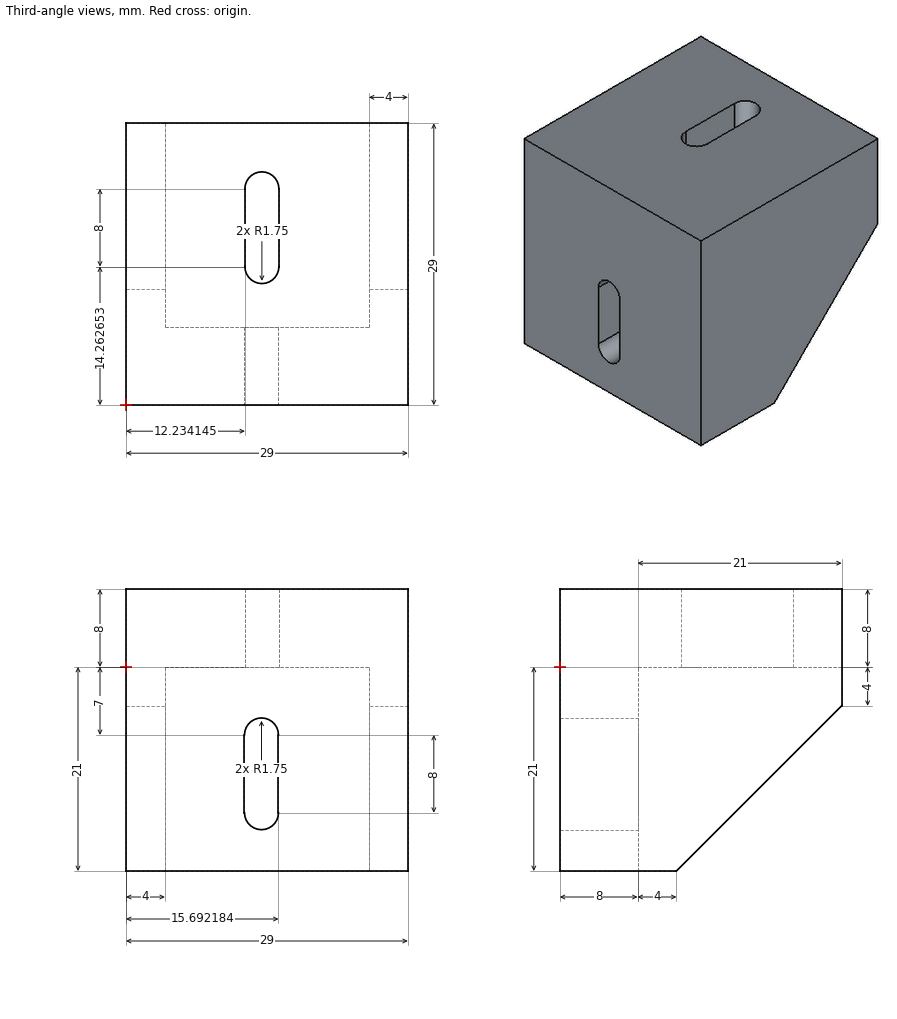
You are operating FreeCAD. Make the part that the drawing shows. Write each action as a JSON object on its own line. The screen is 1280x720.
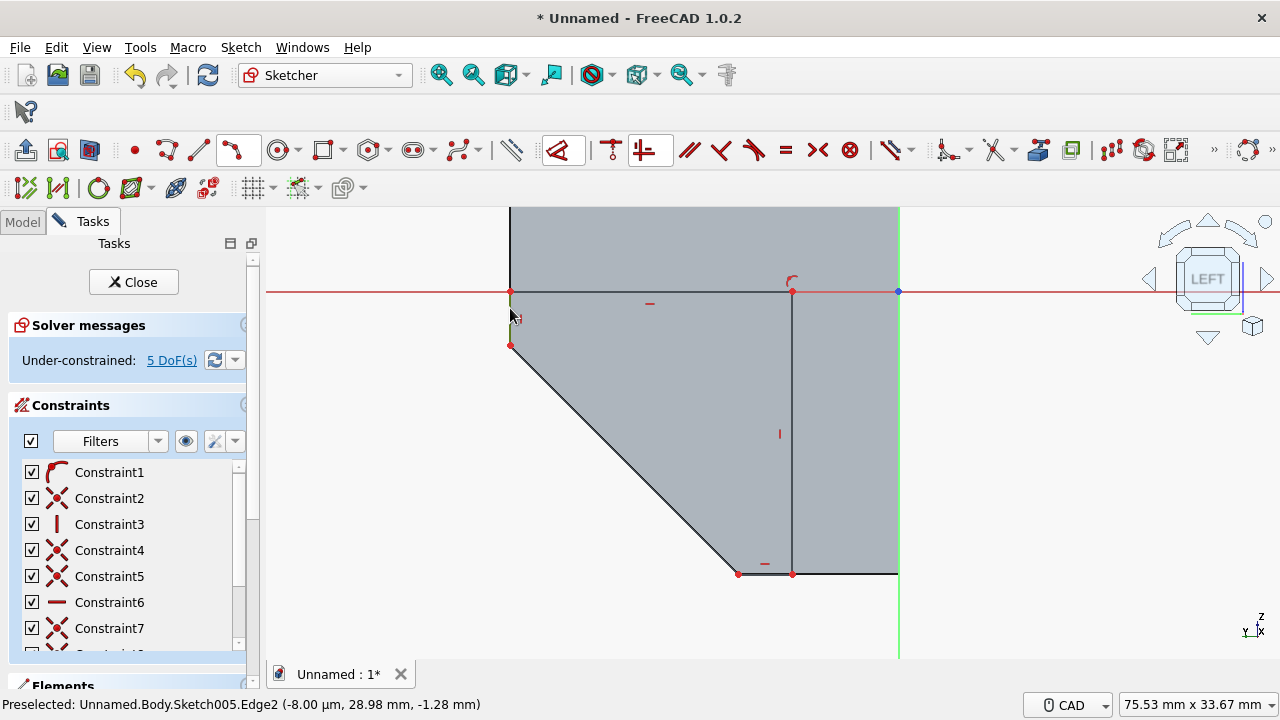
{"action": "key", "text": "i"}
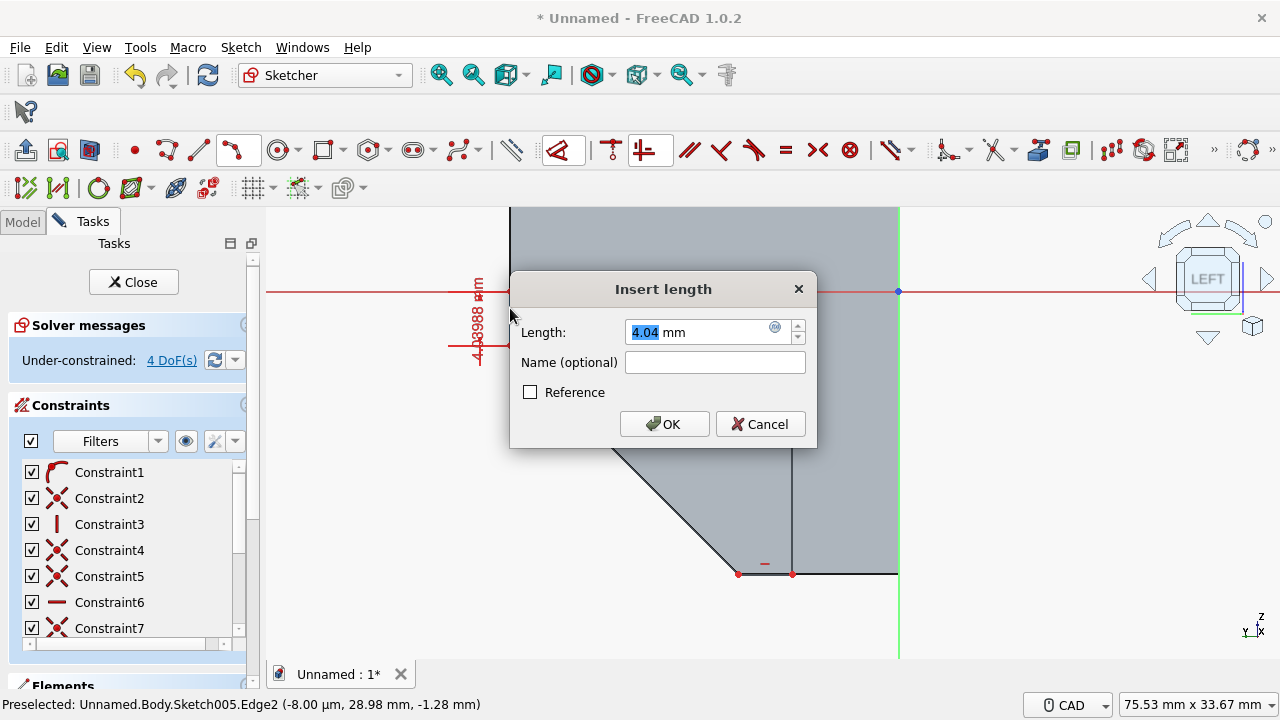
{"action": "type", "text": "4"}
{"action": "key", "text": "Return"}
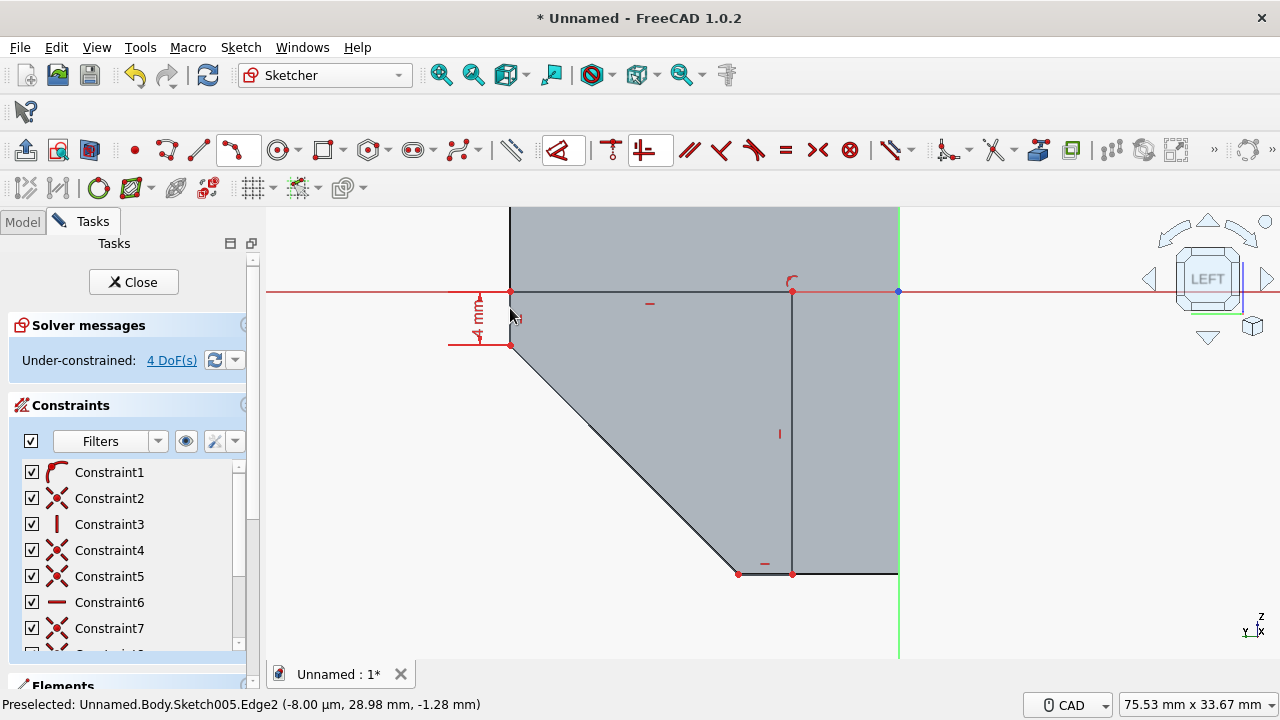
{"action": "left_click", "coordinate": [754, 575]}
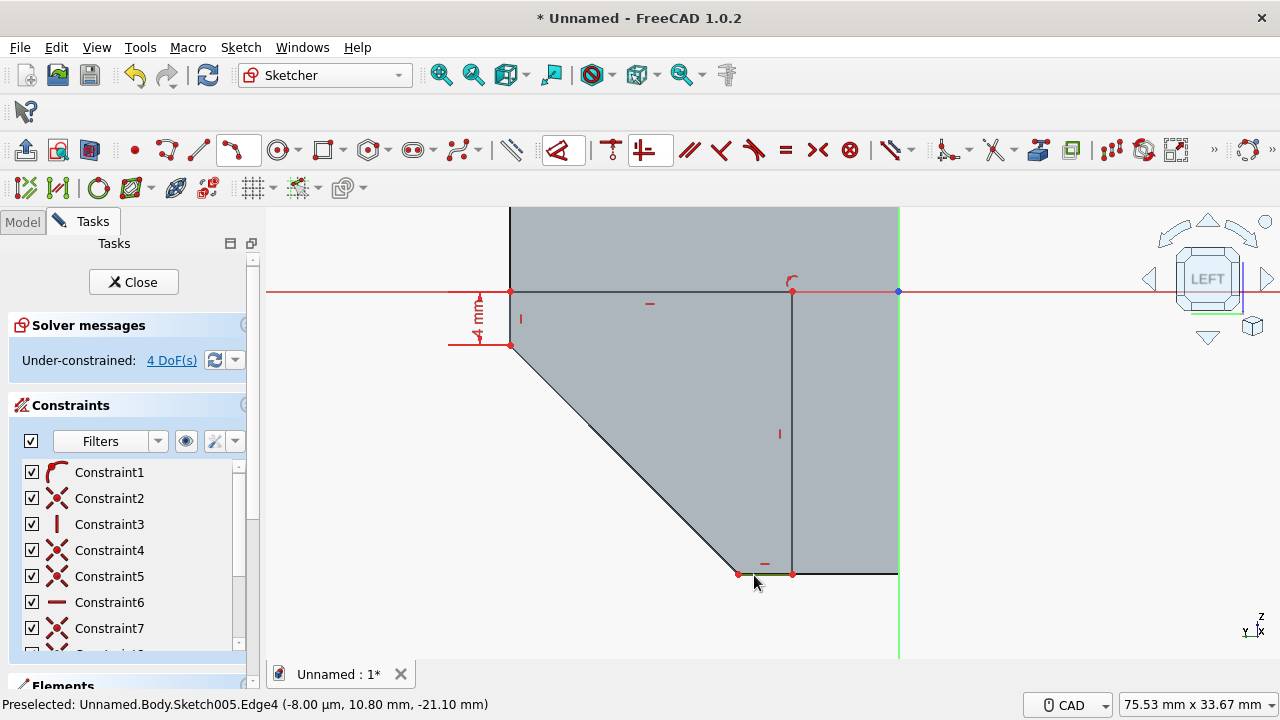
{"action": "left_click", "coordinate": [580, 150]}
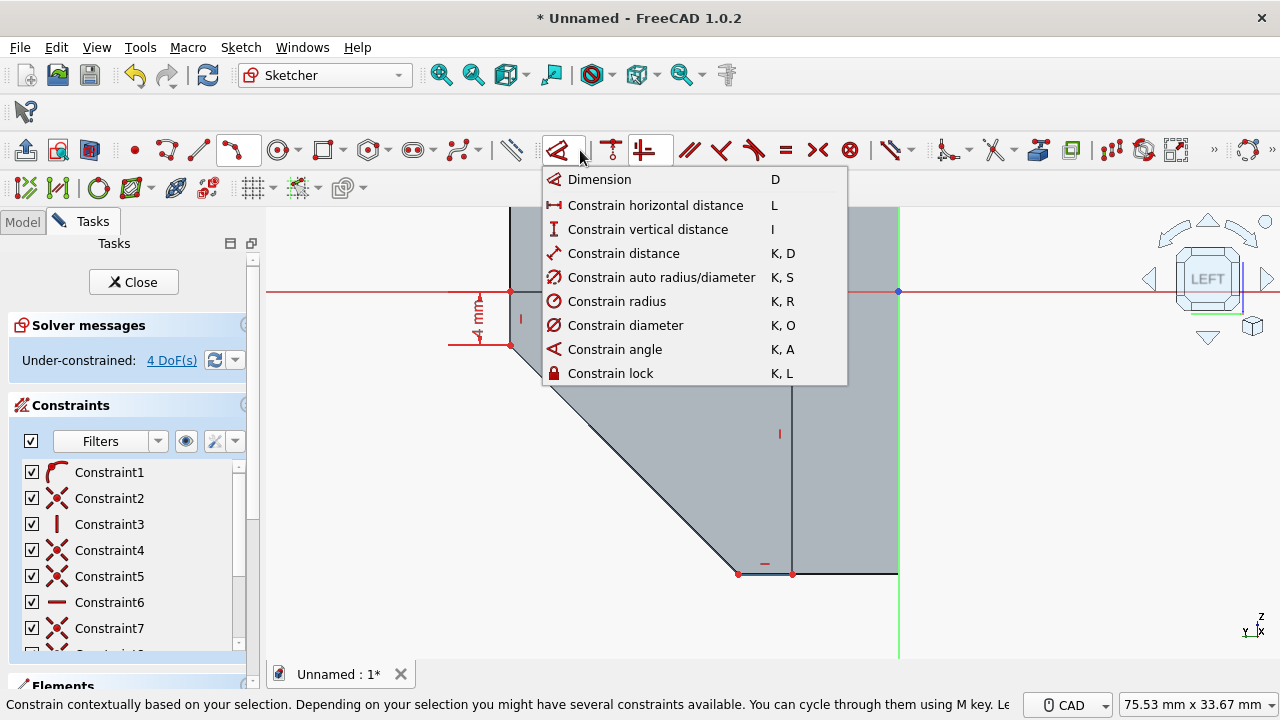
{"action": "left_click", "coordinate": [695, 205]}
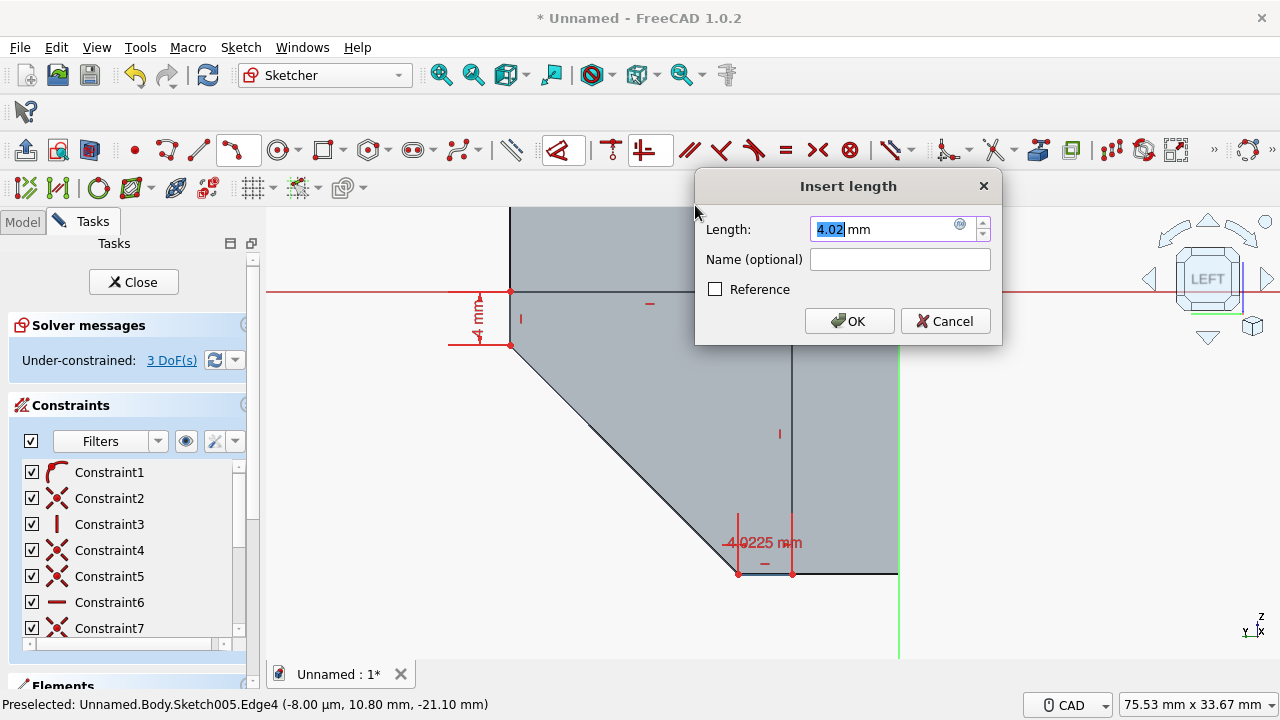
{"action": "type", "text": "4"}
{"action": "key", "text": "Return"}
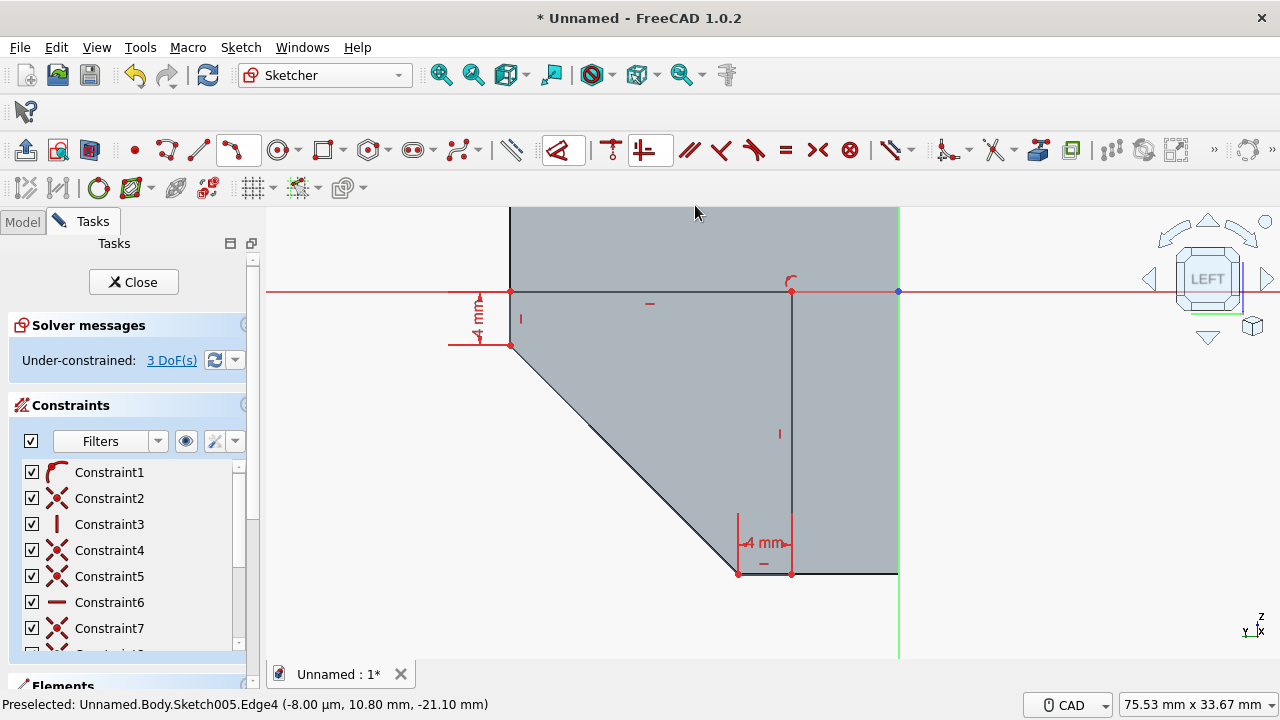
{"action": "left_click", "coordinate": [707, 292]}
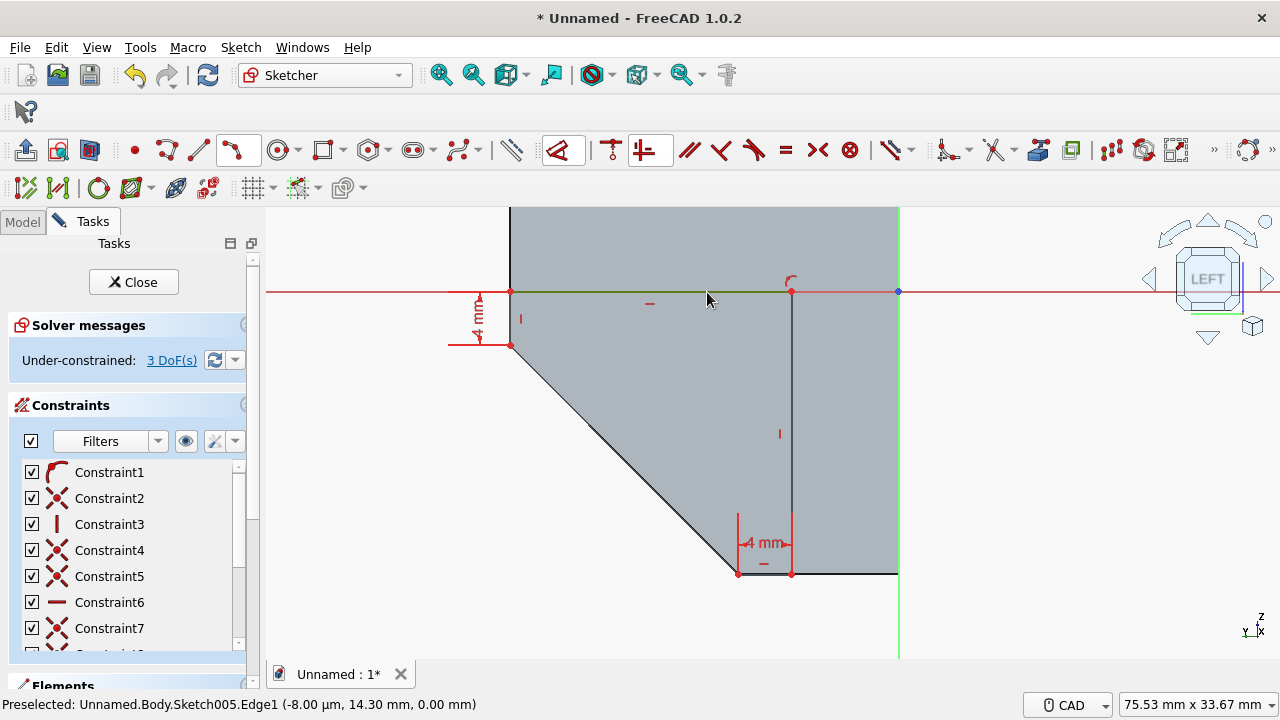
{"action": "key", "text": "l"}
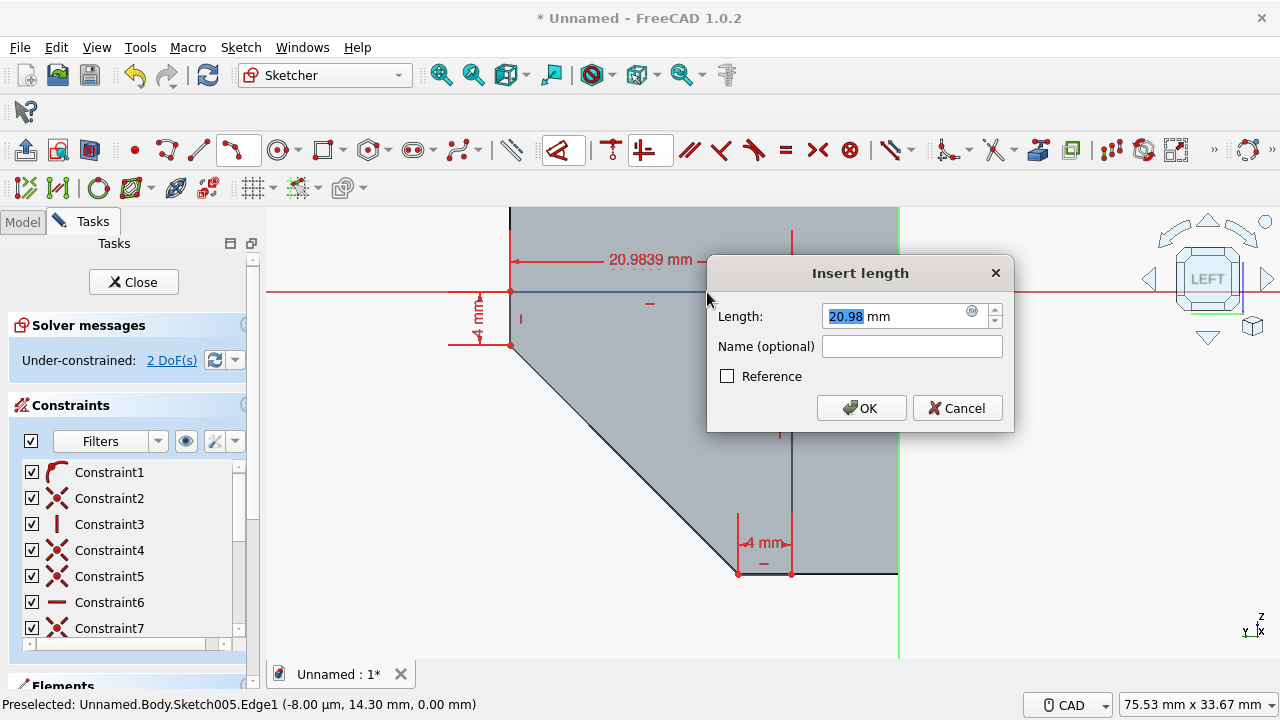
{"action": "type", "text": "21"}
{"action": "key", "text": "Return"}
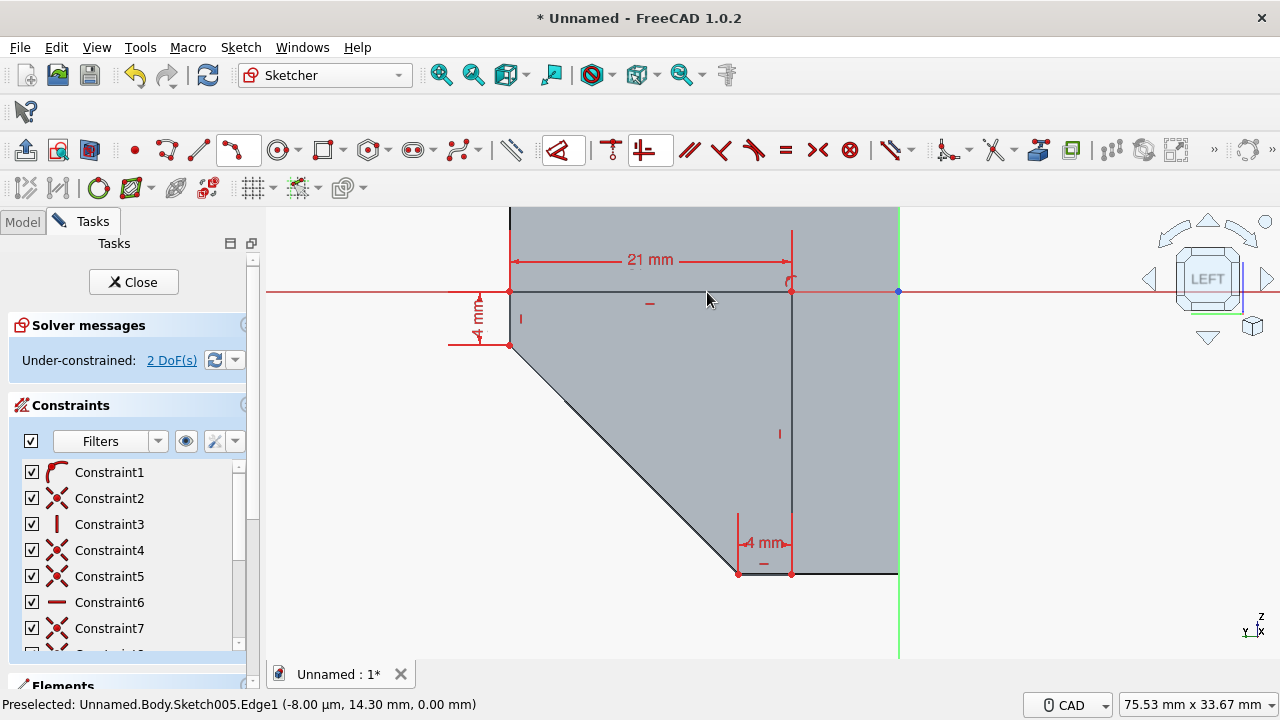
{"action": "left_click", "coordinate": [792, 490]}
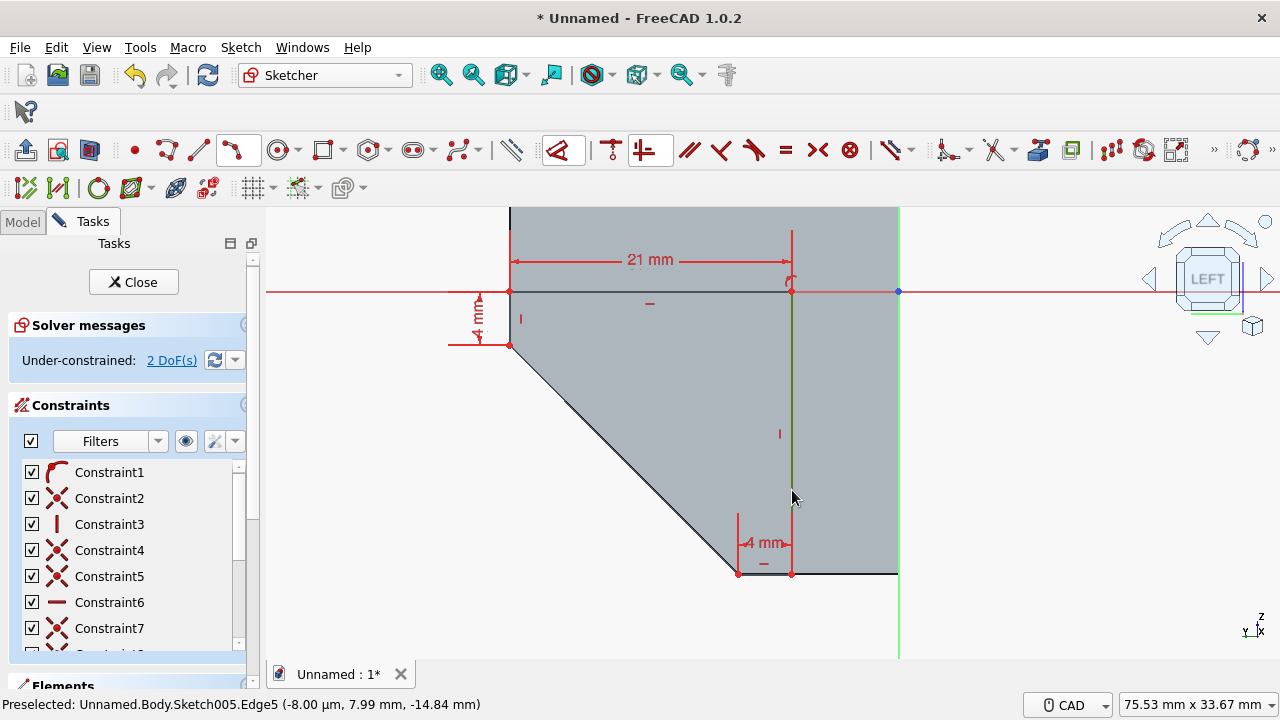
{"action": "left_click", "coordinate": [580, 150]}